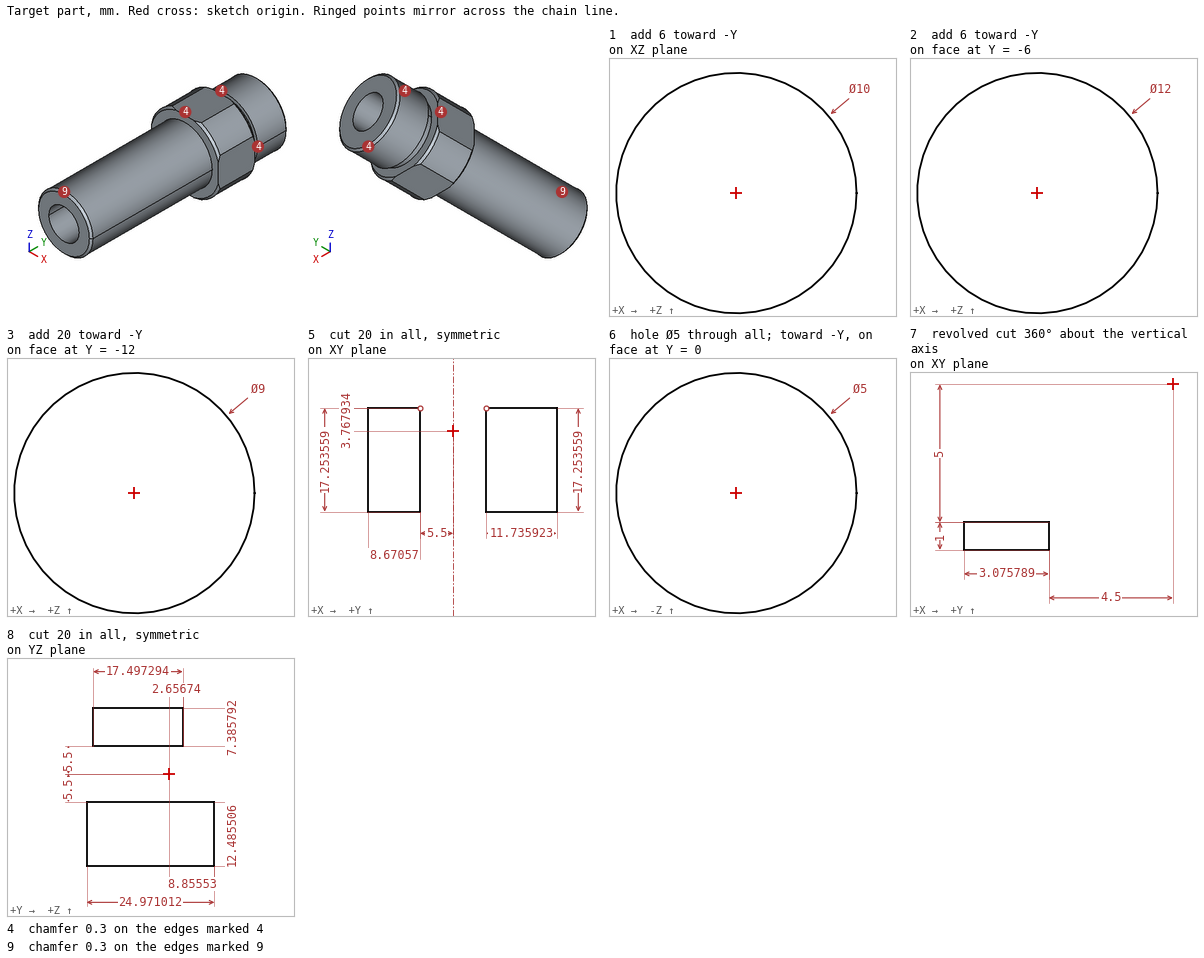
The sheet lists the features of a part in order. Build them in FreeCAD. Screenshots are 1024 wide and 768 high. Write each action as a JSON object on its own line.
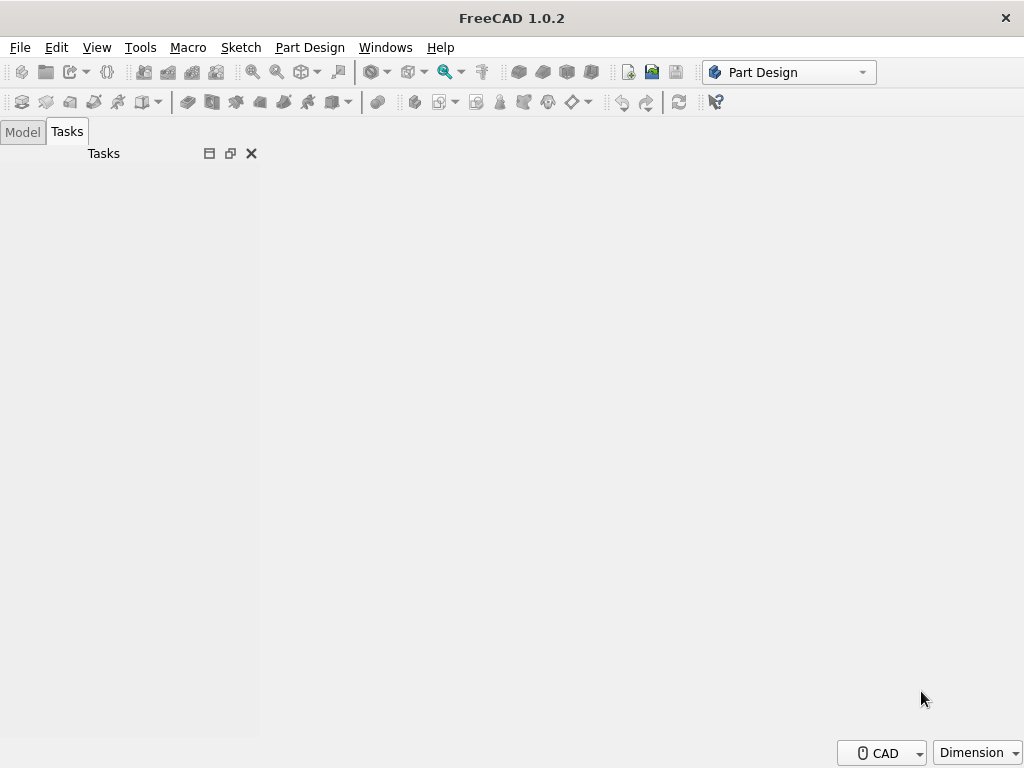
{"action": "key", "text": "ctrl+n"}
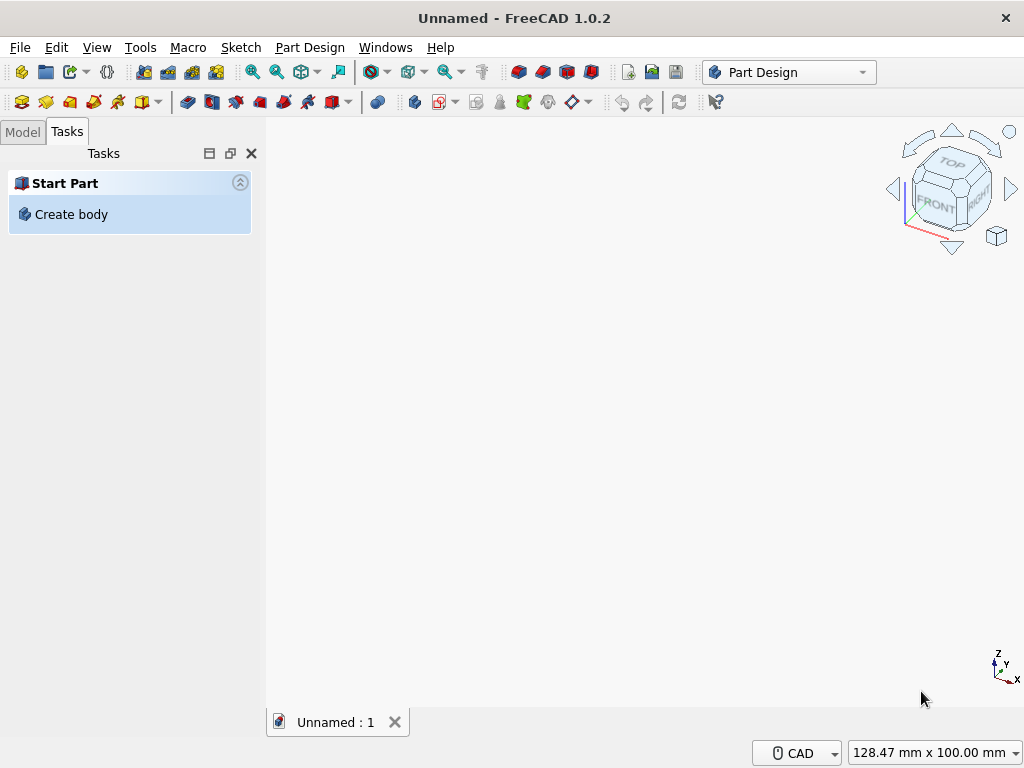
{"action": "left_click", "coordinate": [440, 102]}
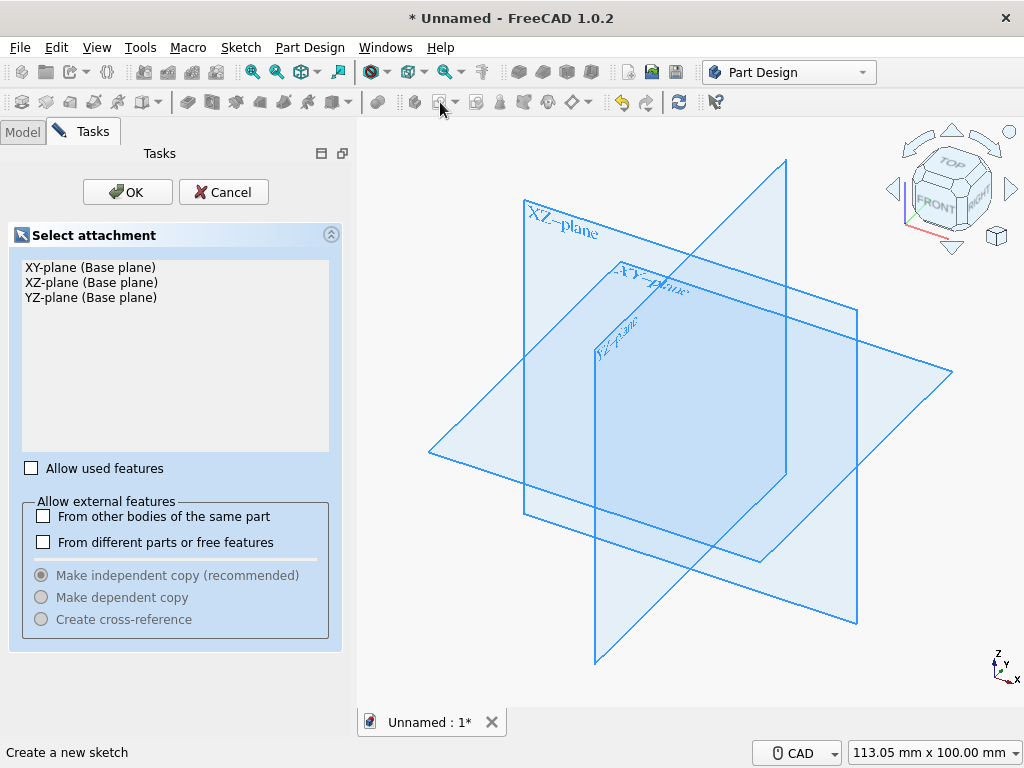
{"action": "left_click", "coordinate": [82, 282]}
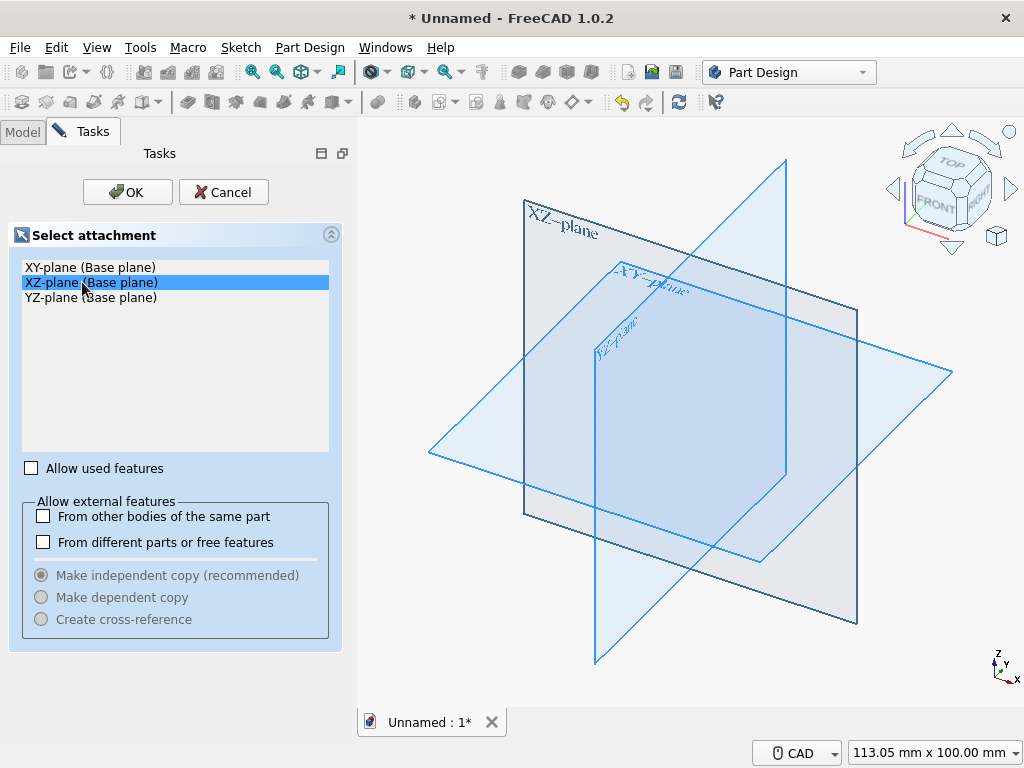
{"action": "left_click", "coordinate": [128, 192]}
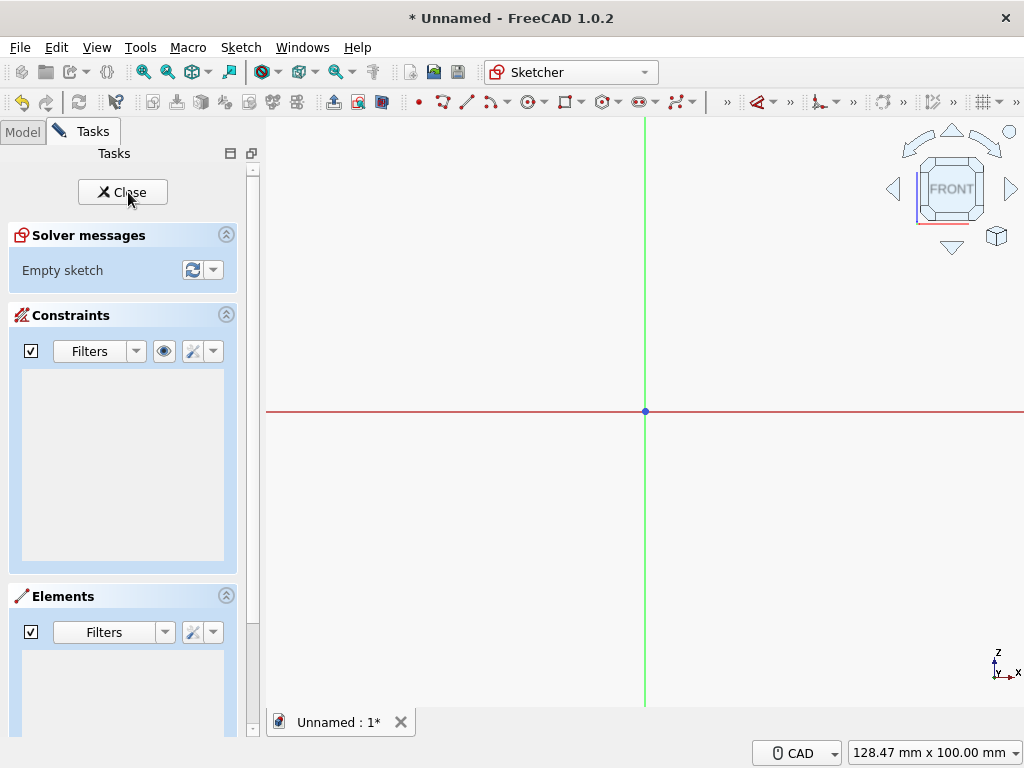
{"action": "scroll", "coordinate": [659, 412], "scroll_direction": "up", "scroll_amount": 9}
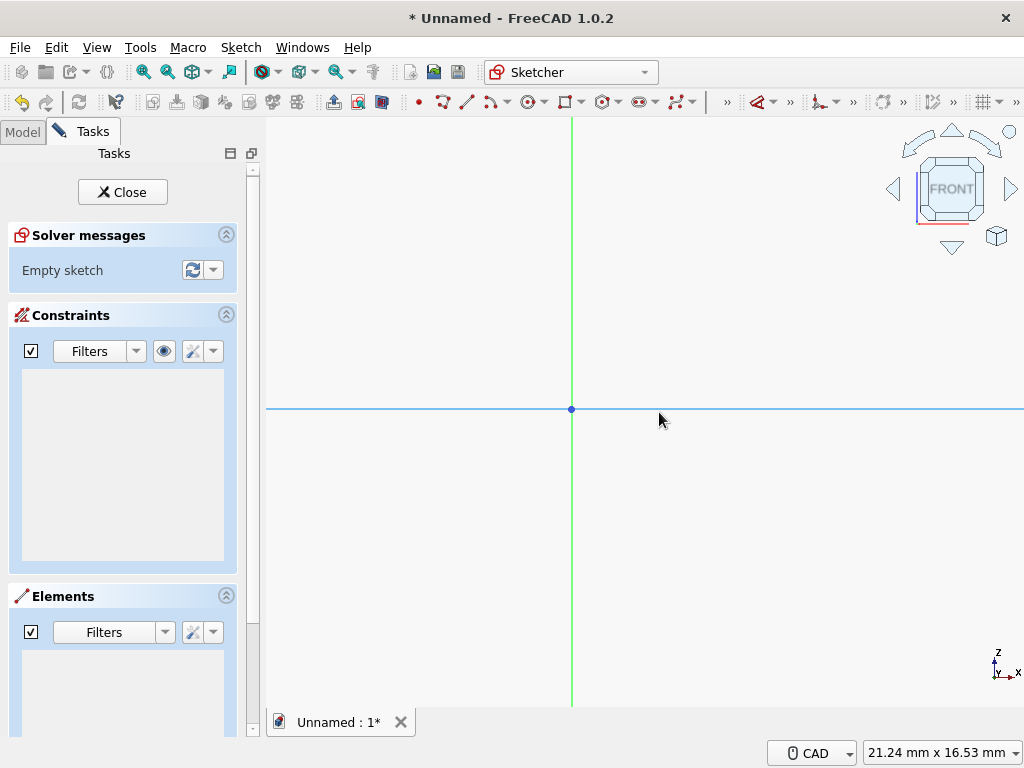
{"action": "key", "text": "g c"}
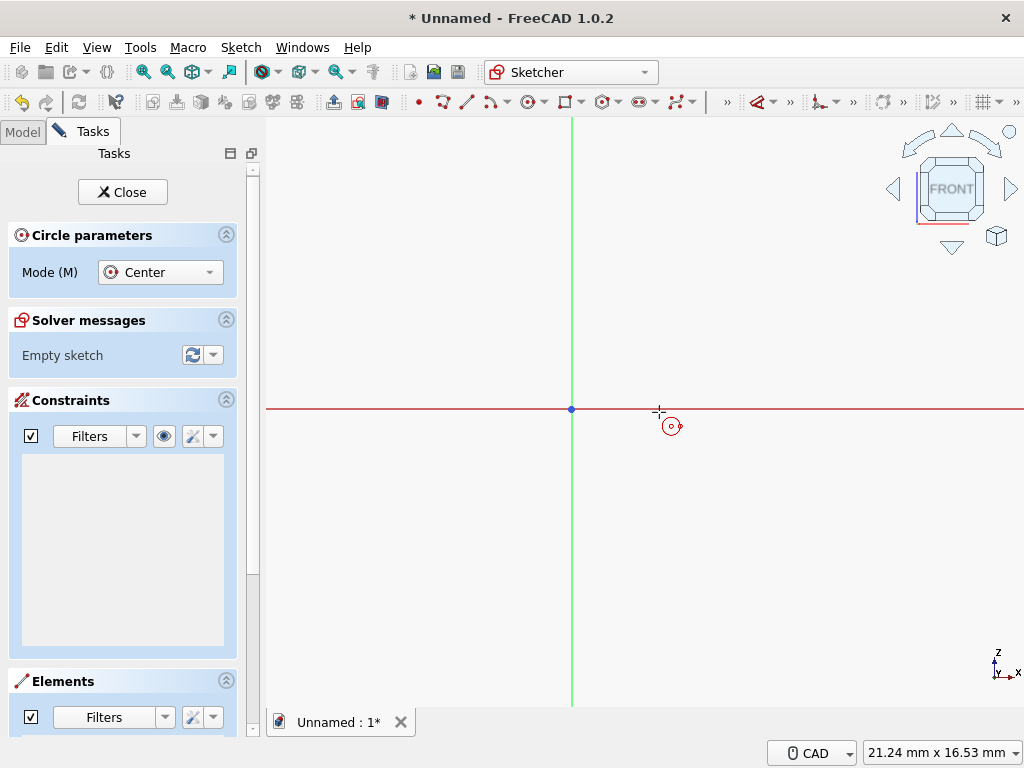
{"action": "left_click", "coordinate": [572, 409]}
{"action": "mouse_move", "coordinate": [698, 283]}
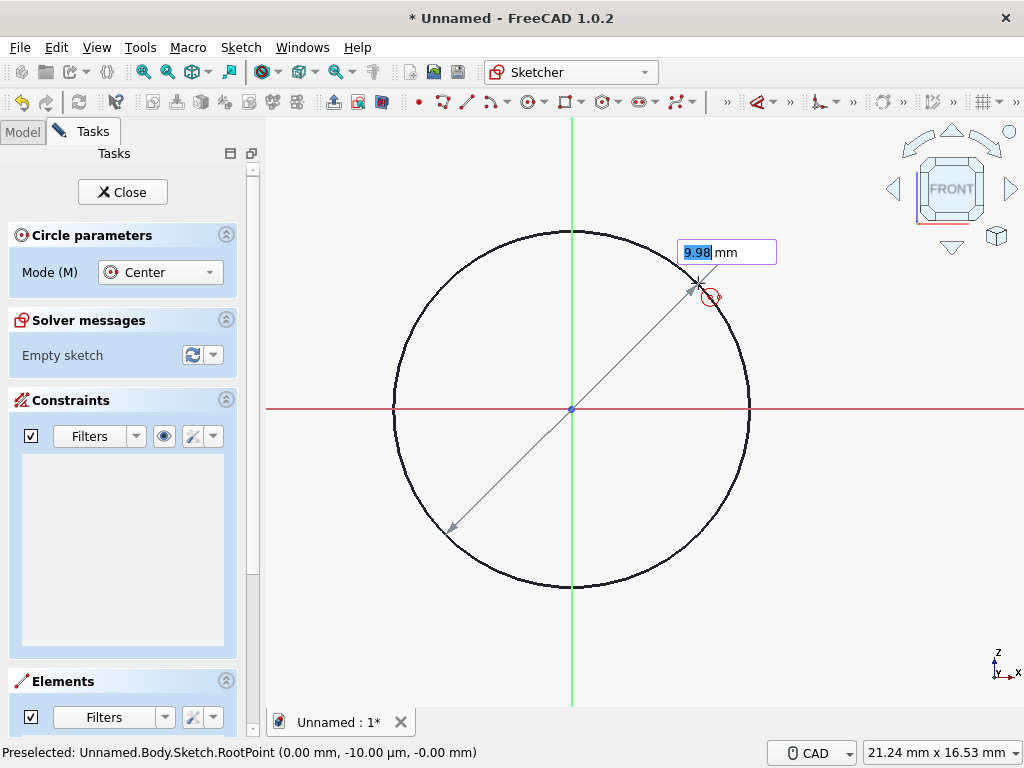
{"action": "type", "text": "10"}
{"action": "key", "text": "Return"}
{"action": "key", "text": "Escape"}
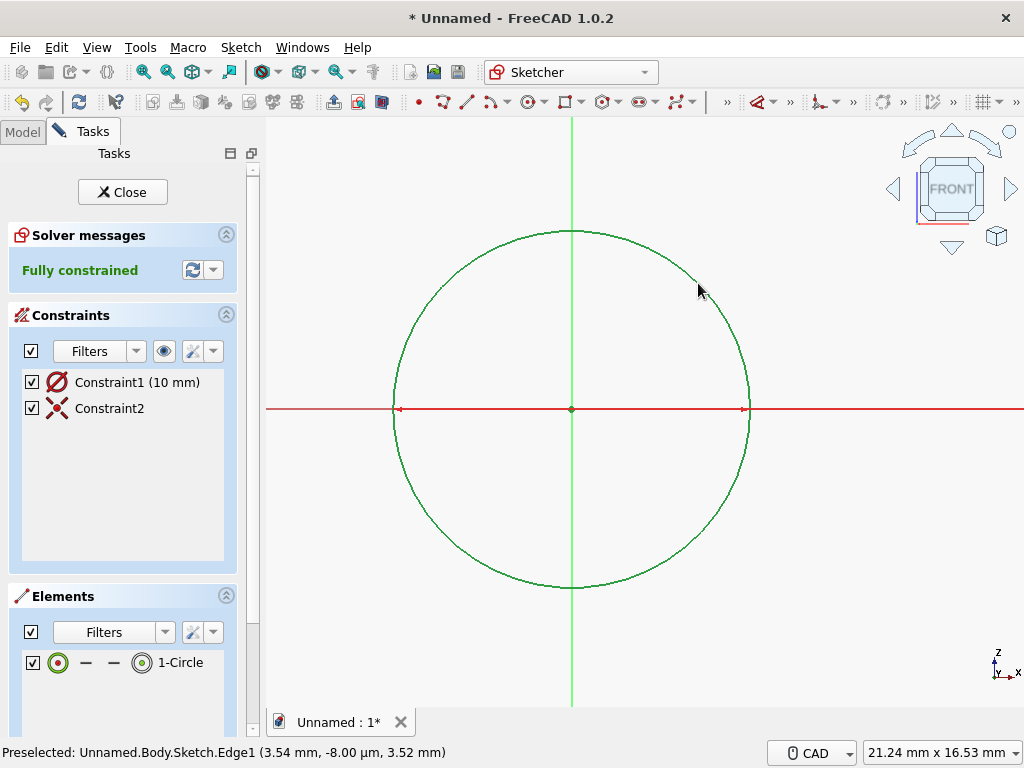
{"action": "left_click", "coordinate": [123, 192]}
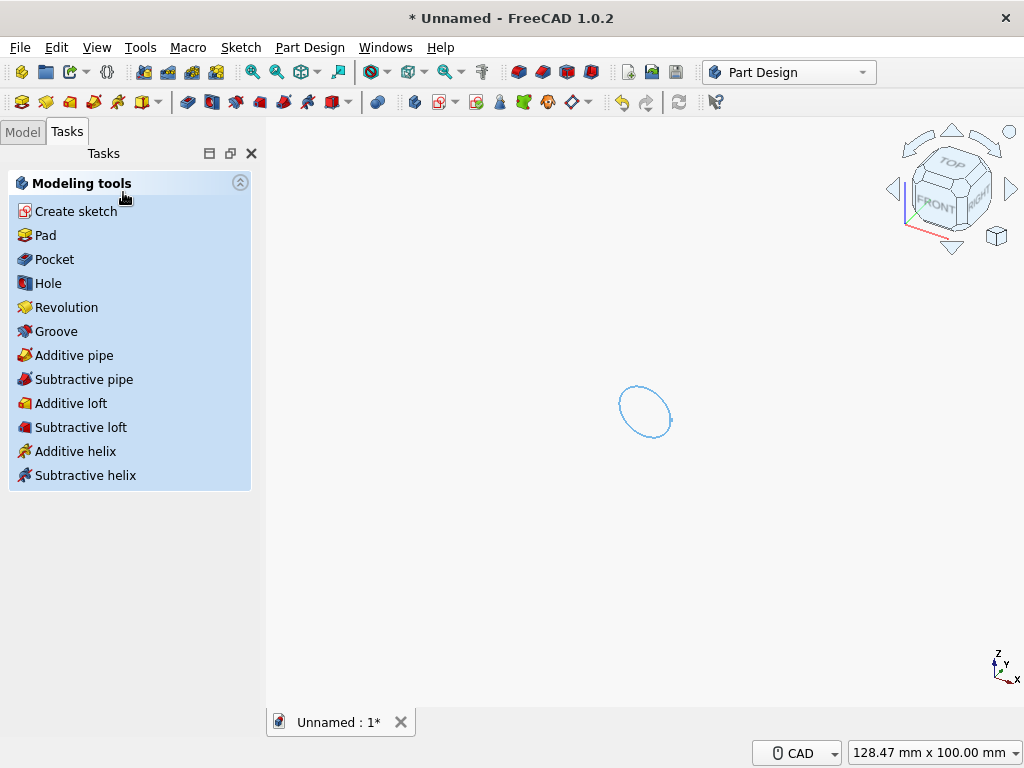
{"action": "left_click", "coordinate": [22, 102]}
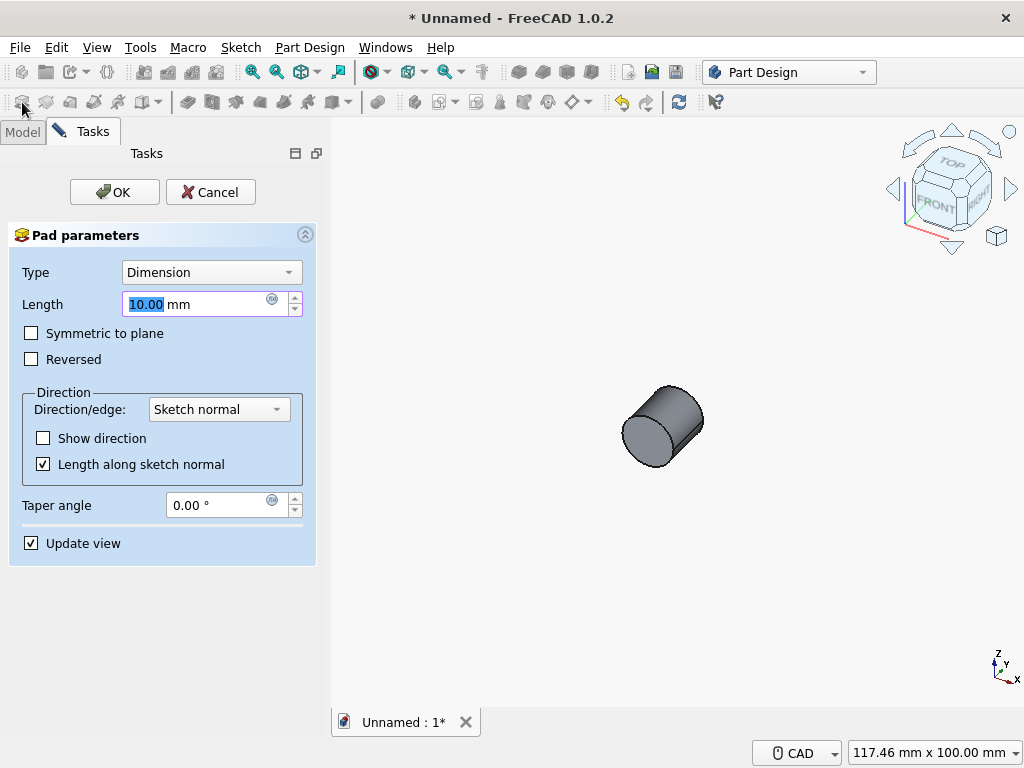
{"action": "type", "text": "6"}
{"action": "key", "text": "Tab"}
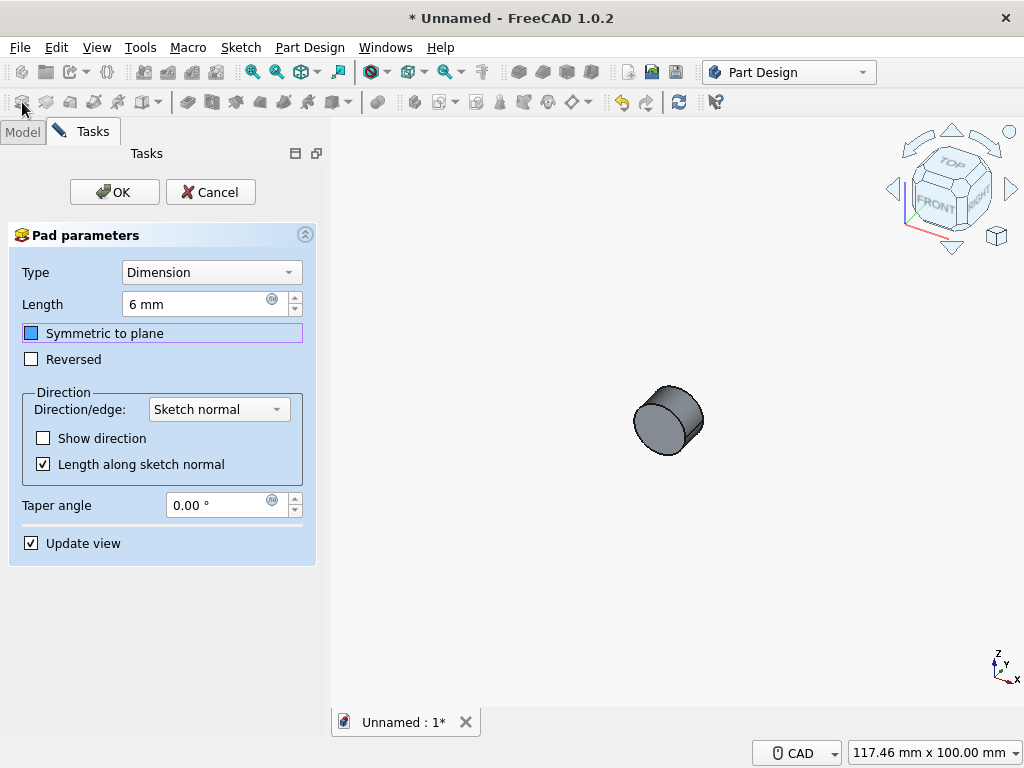
{"action": "left_click", "coordinate": [115, 192]}